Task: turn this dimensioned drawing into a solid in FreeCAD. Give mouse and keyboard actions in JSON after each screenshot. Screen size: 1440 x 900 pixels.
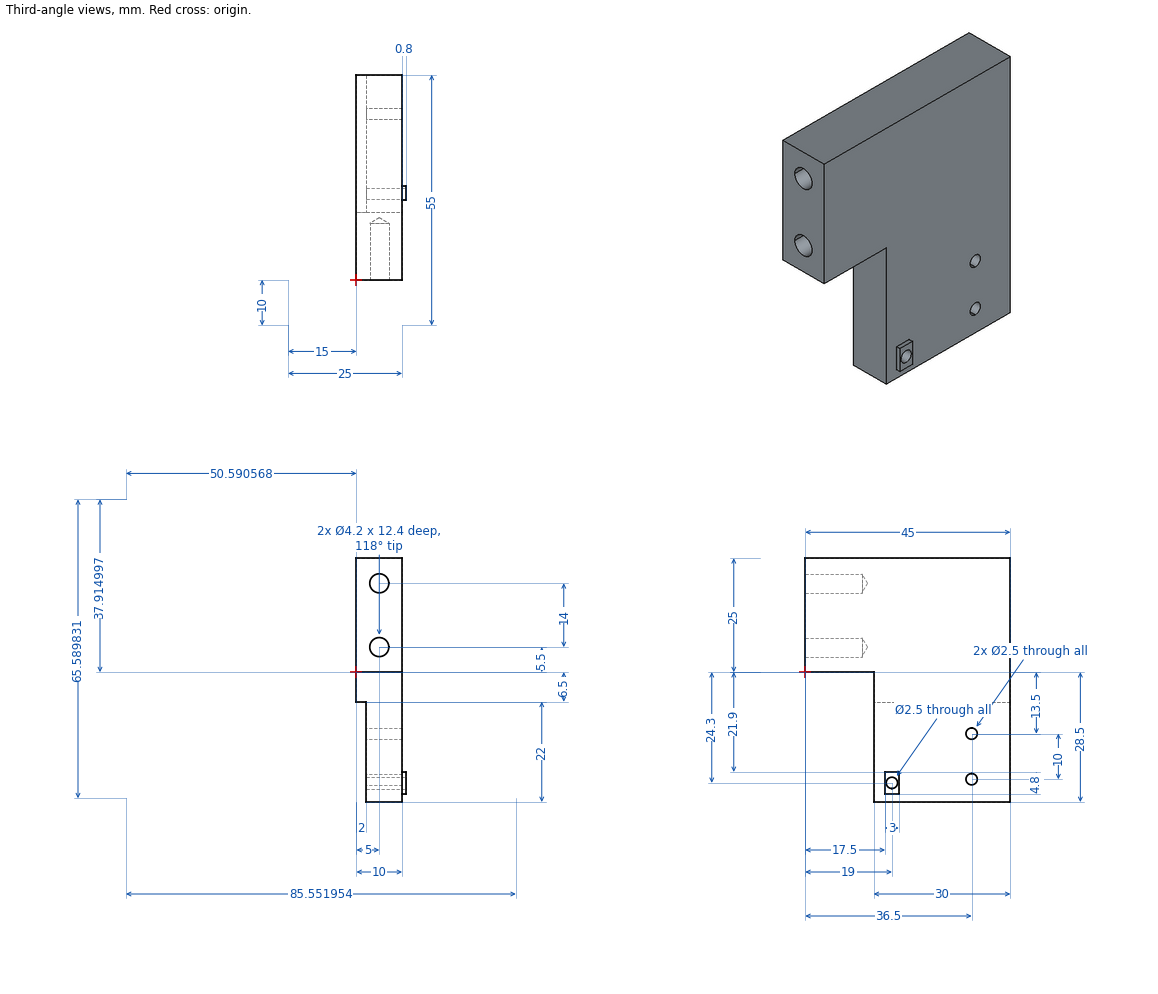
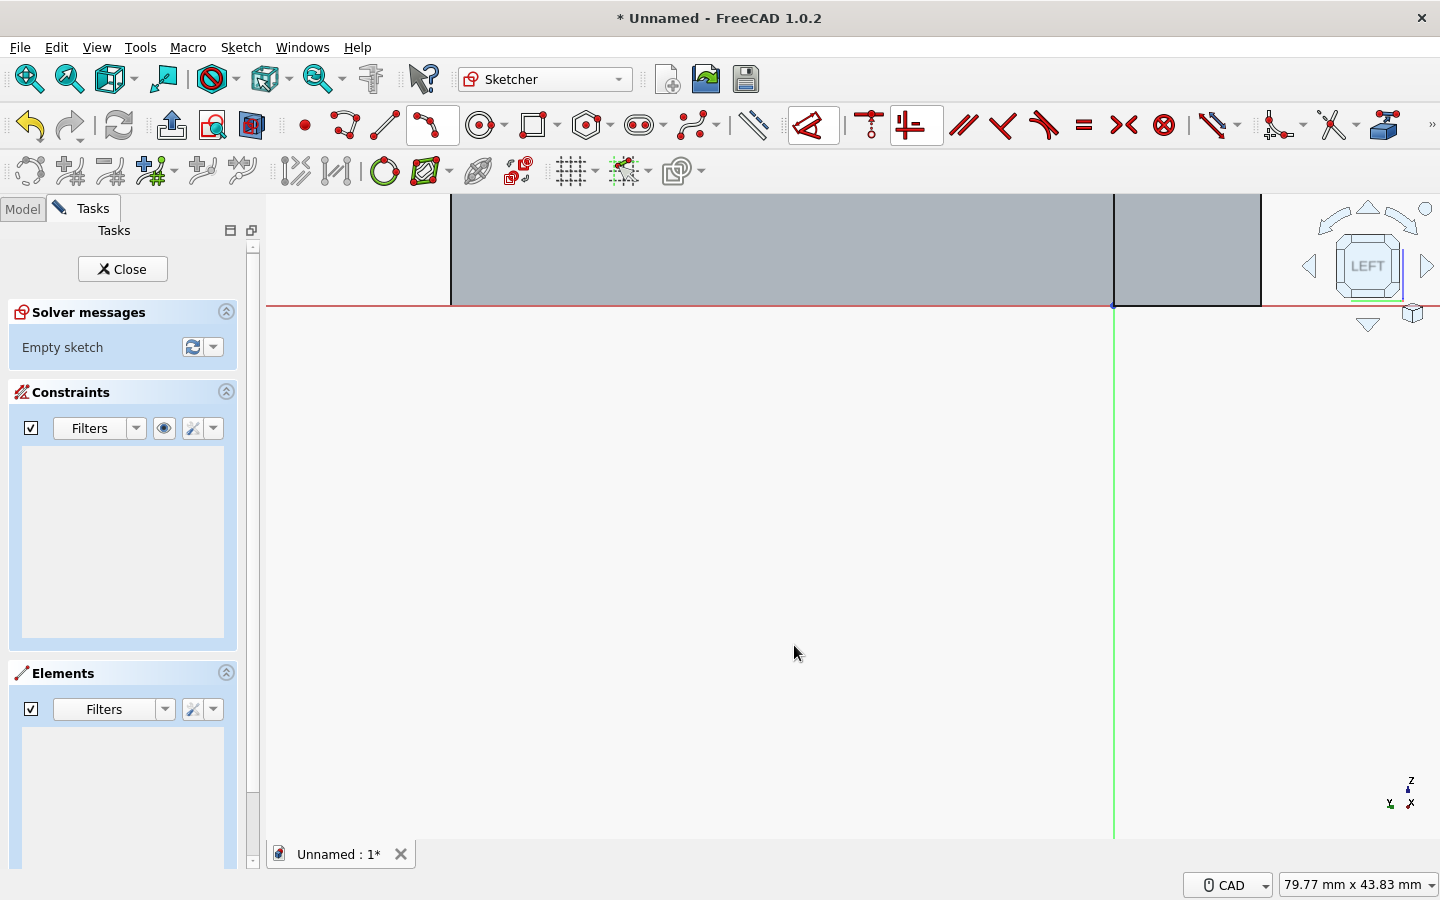
{"action": "left_click", "coordinate": [534, 126]}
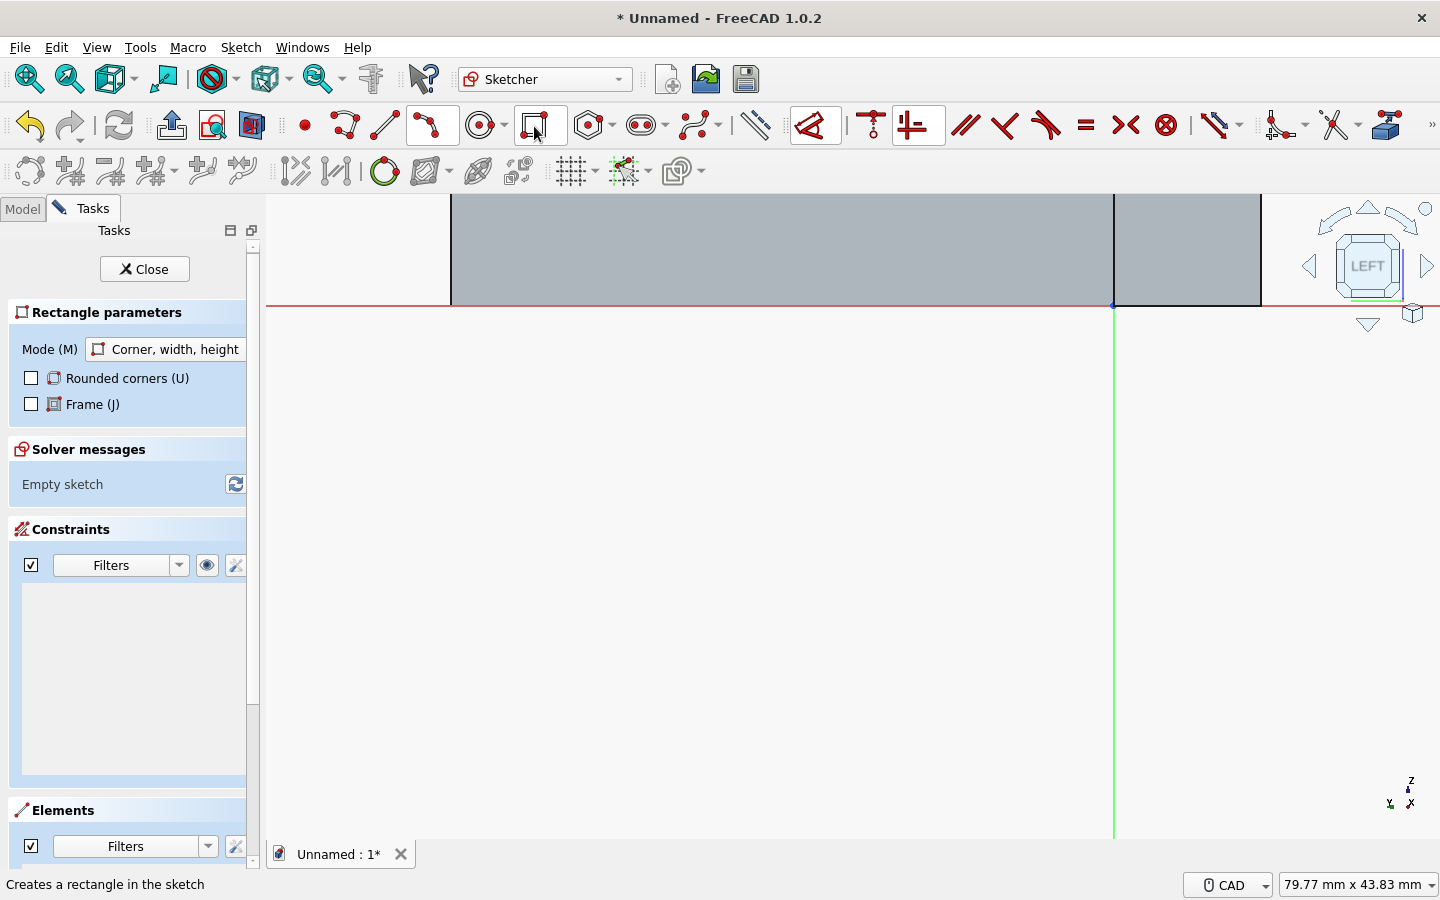
{"action": "left_click", "coordinate": [451, 306]}
{"action": "left_click", "coordinate": [893, 725]}
{"action": "key", "text": "Escape"}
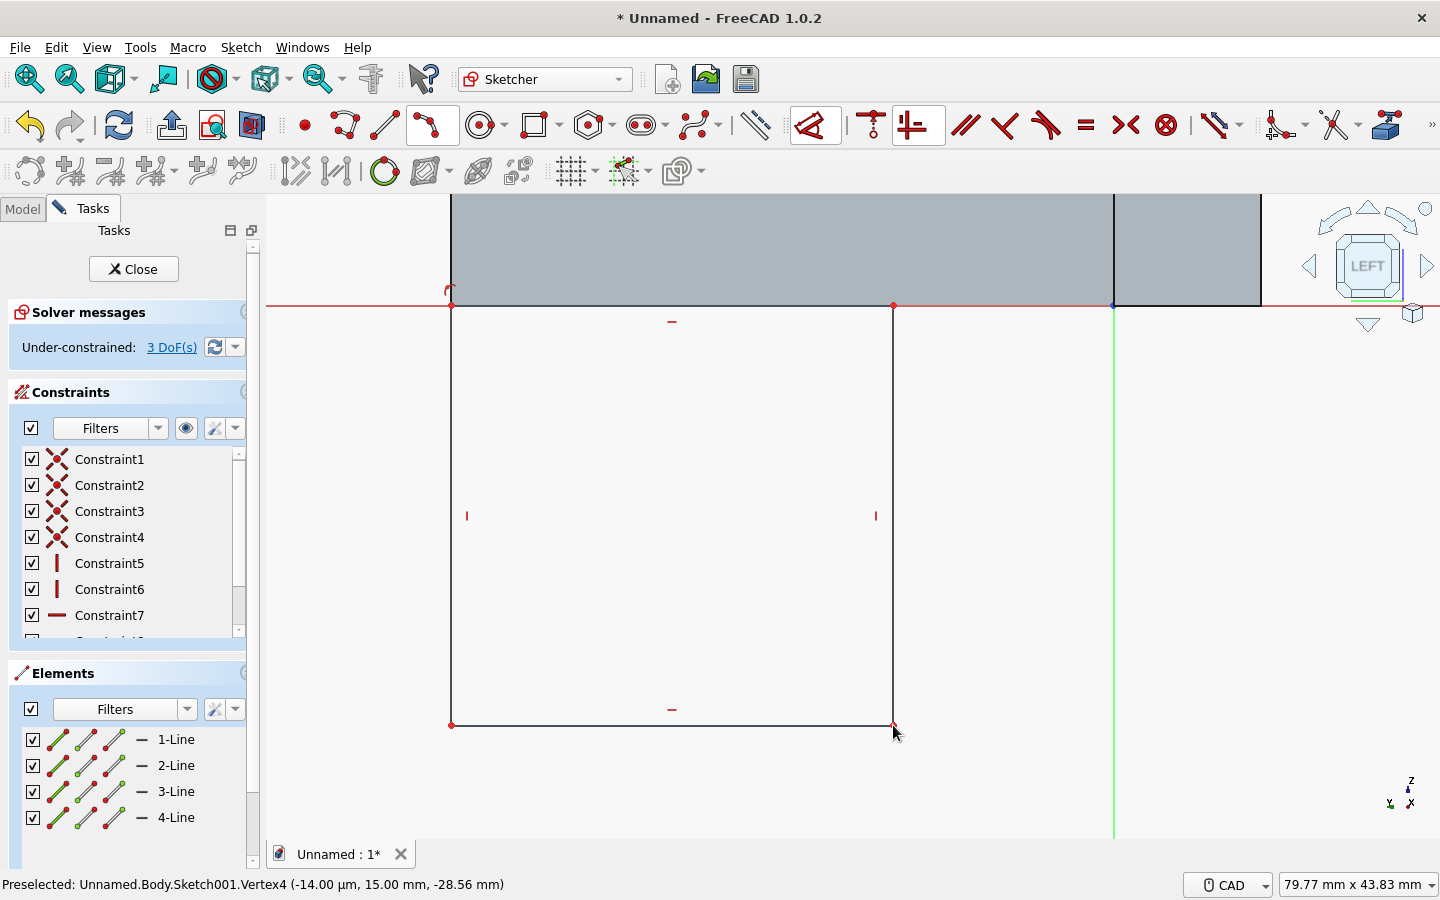
{"action": "left_click", "coordinate": [584, 726]}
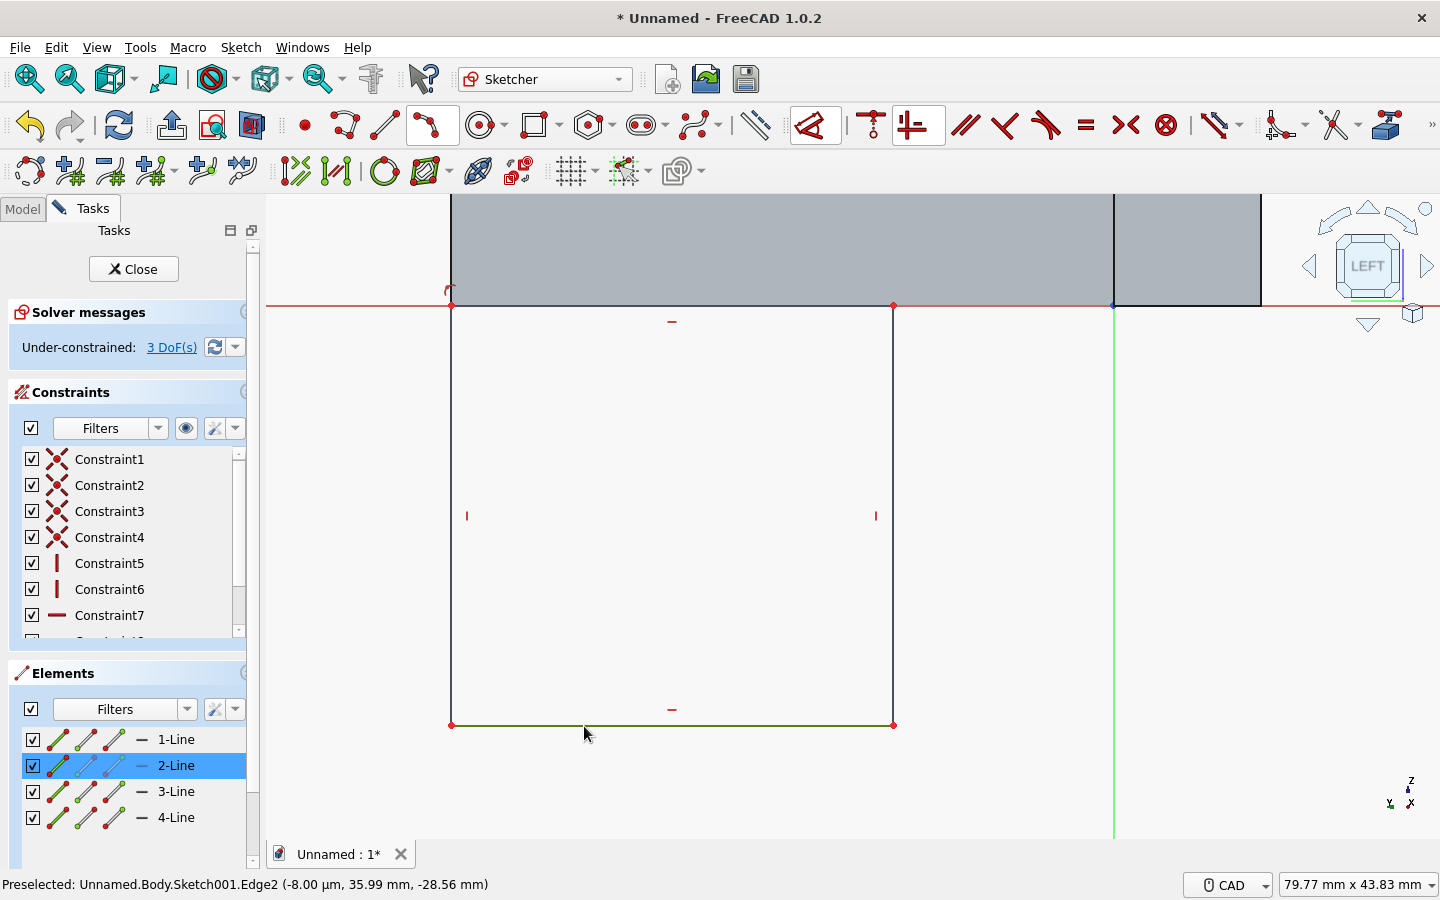
{"action": "left_click", "coordinate": [836, 126]}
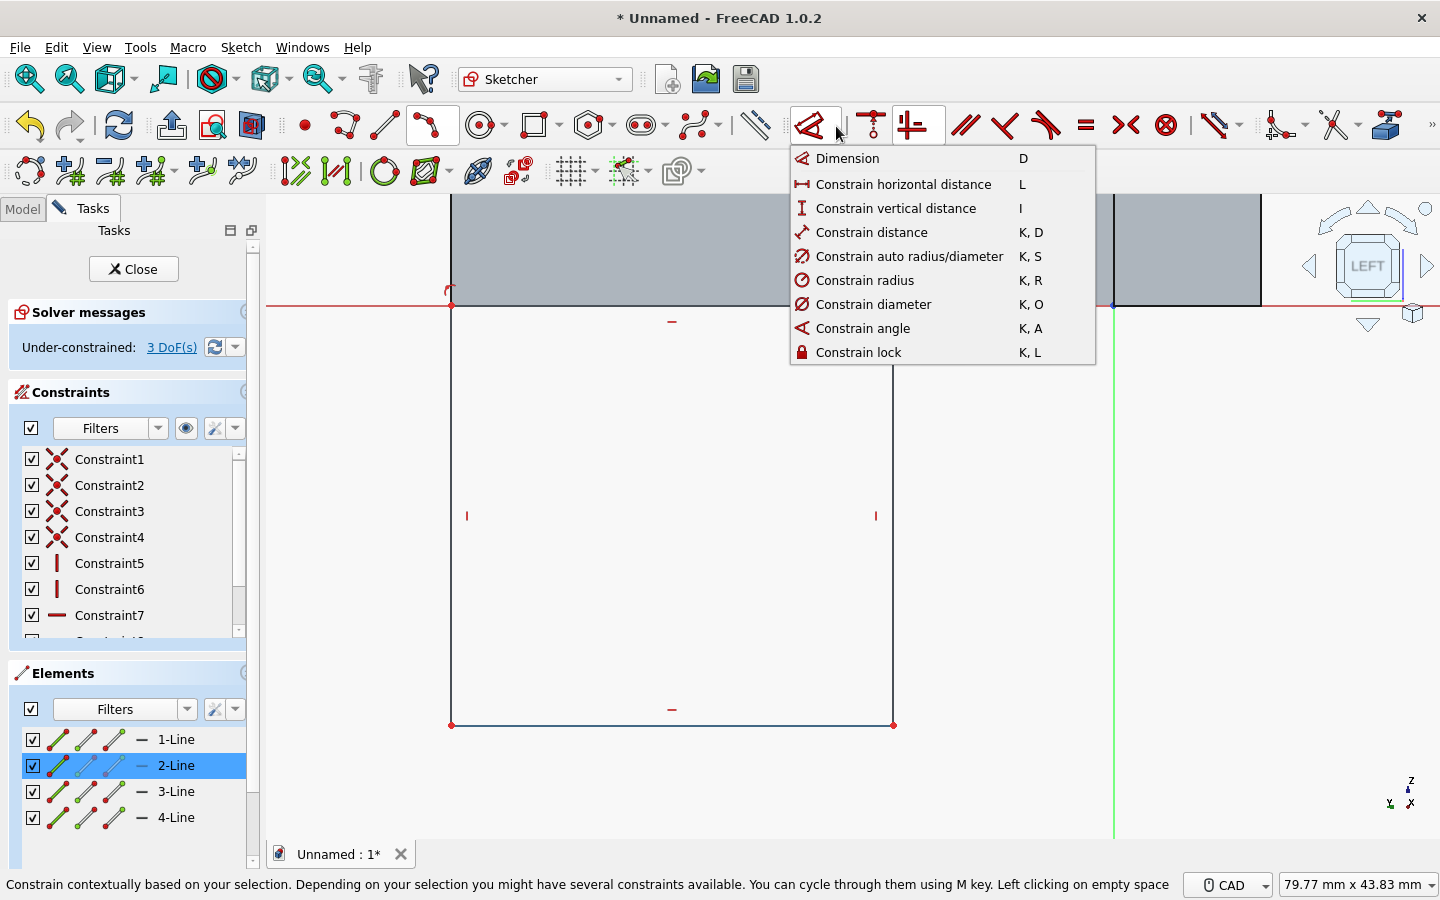
{"action": "left_click", "coordinate": [943, 184]}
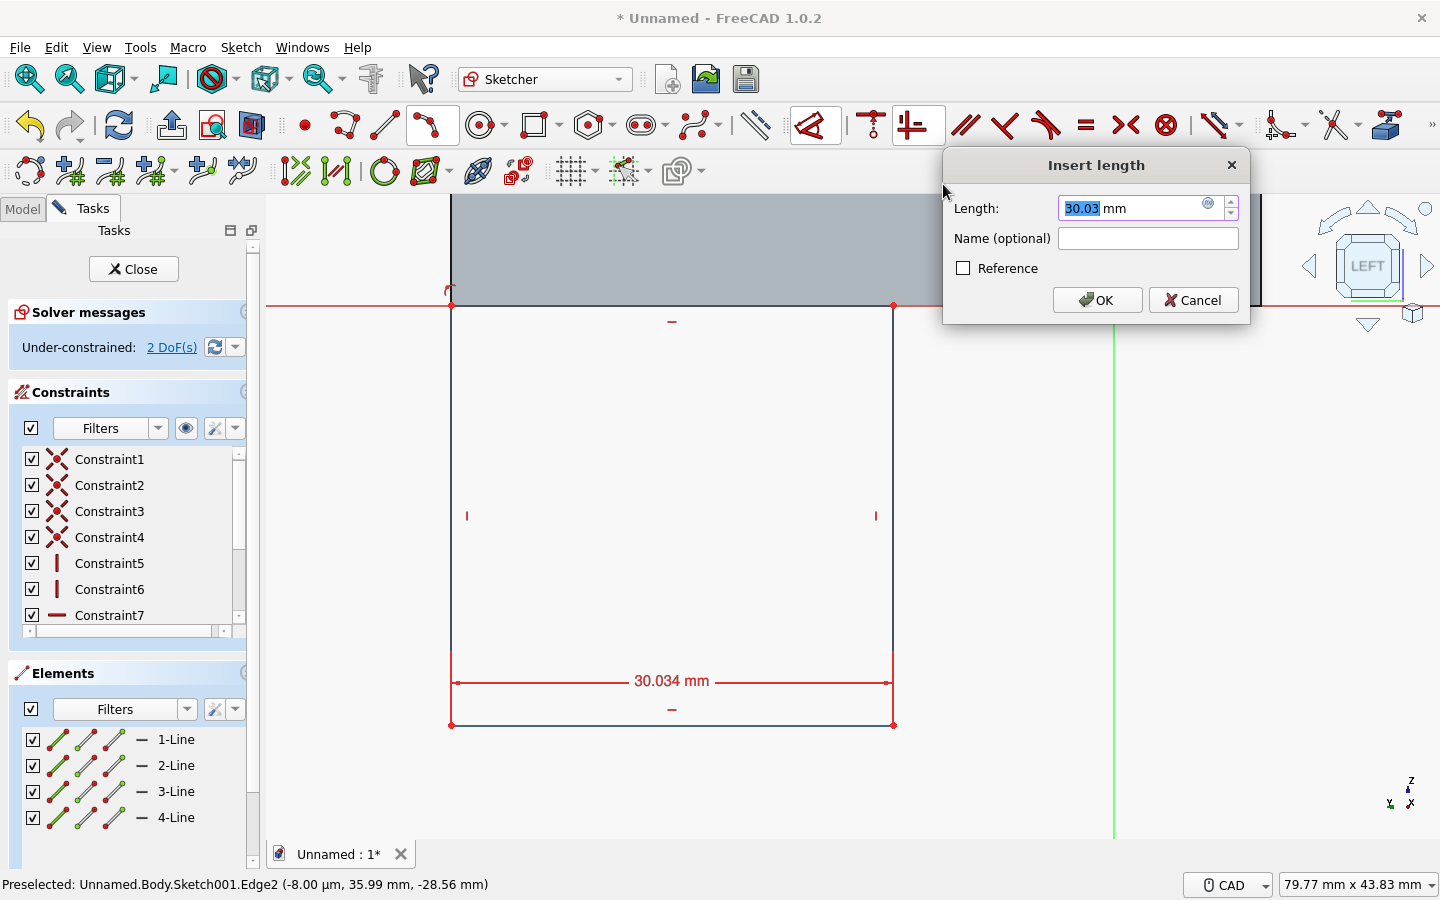
{"action": "type", "text": "30"}
{"action": "key", "text": "Return"}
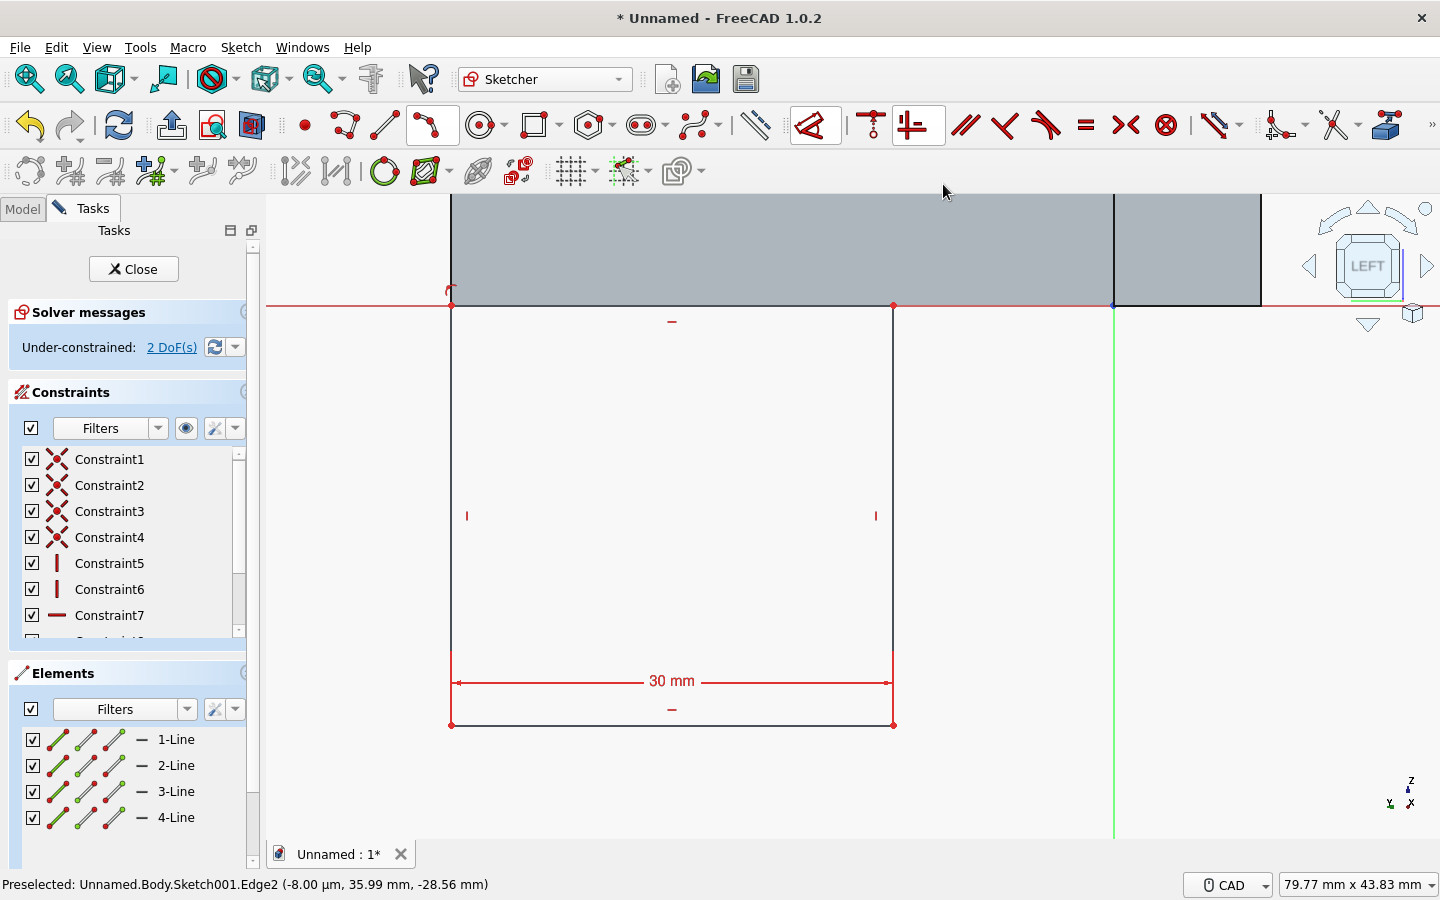
{"action": "left_click", "coordinate": [452, 306]}